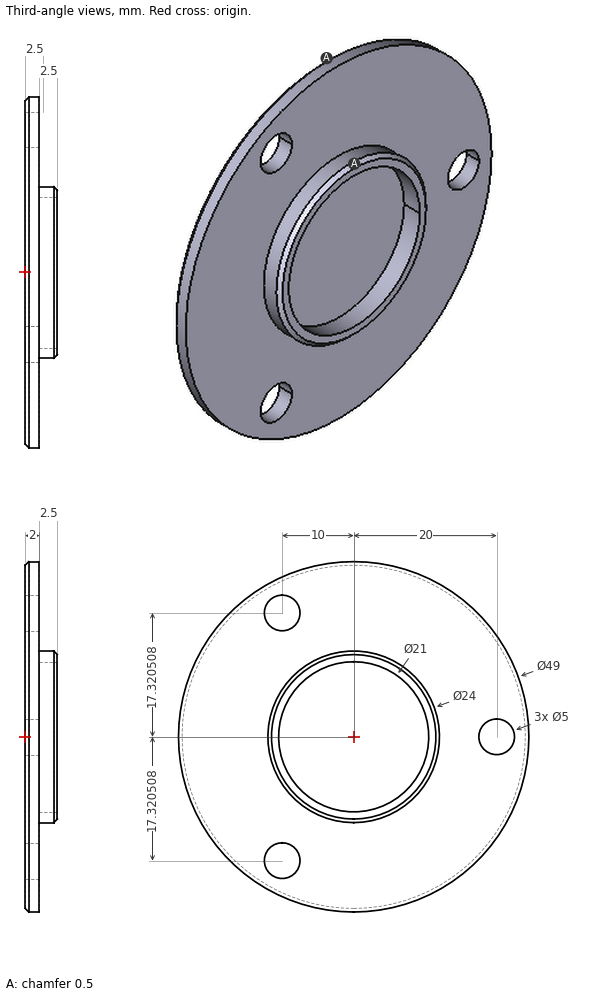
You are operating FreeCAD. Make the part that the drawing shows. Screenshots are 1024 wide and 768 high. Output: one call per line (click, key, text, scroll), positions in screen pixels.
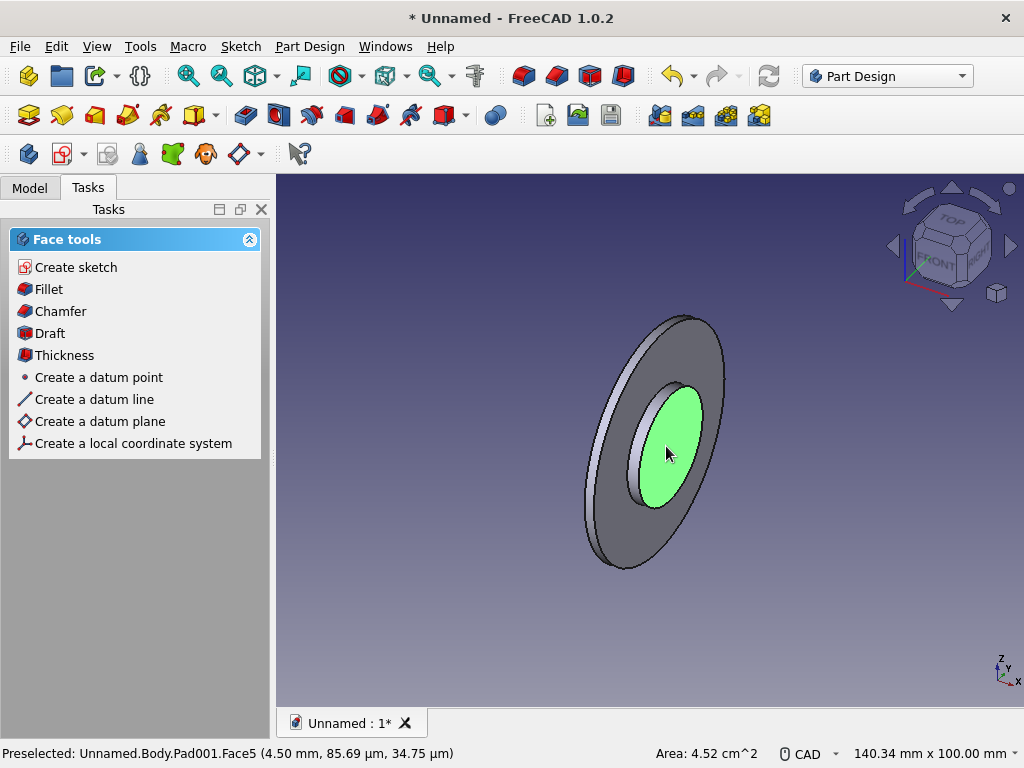
click(62, 154)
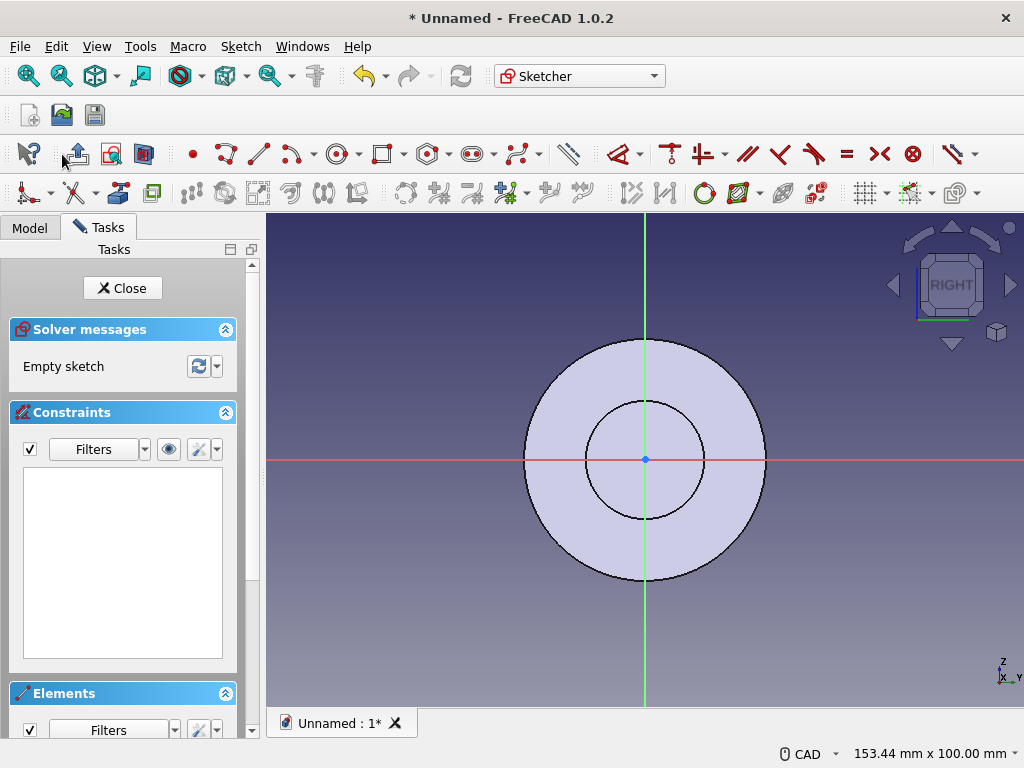
scroll(685, 460, up, 5)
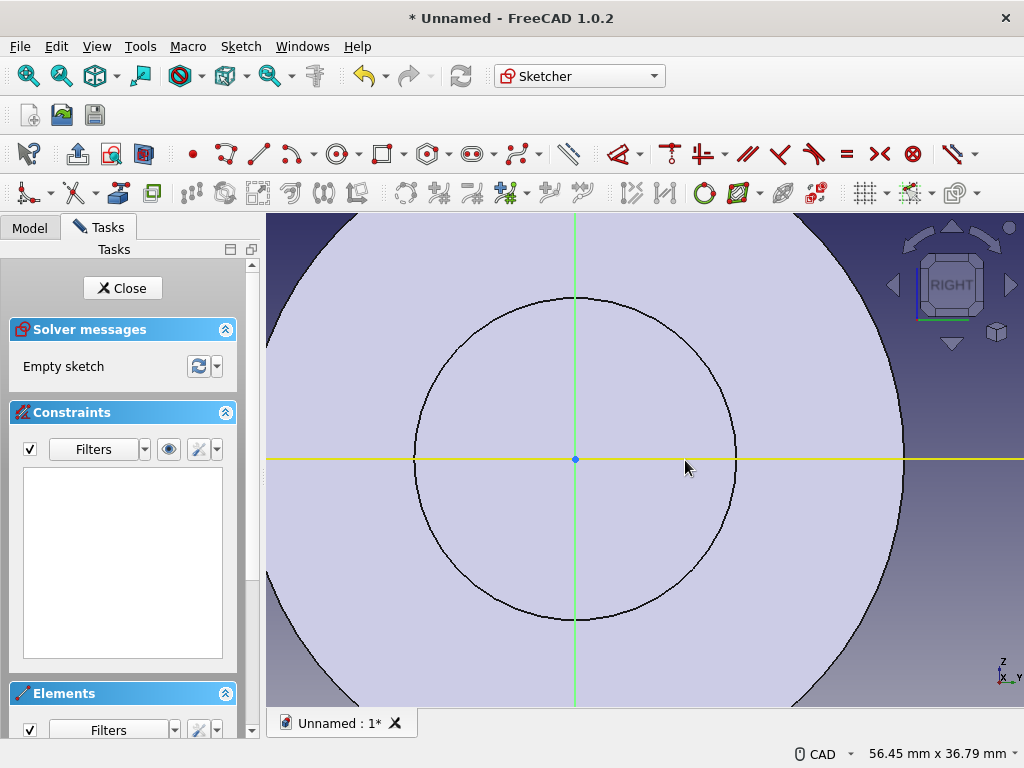
click(336, 154)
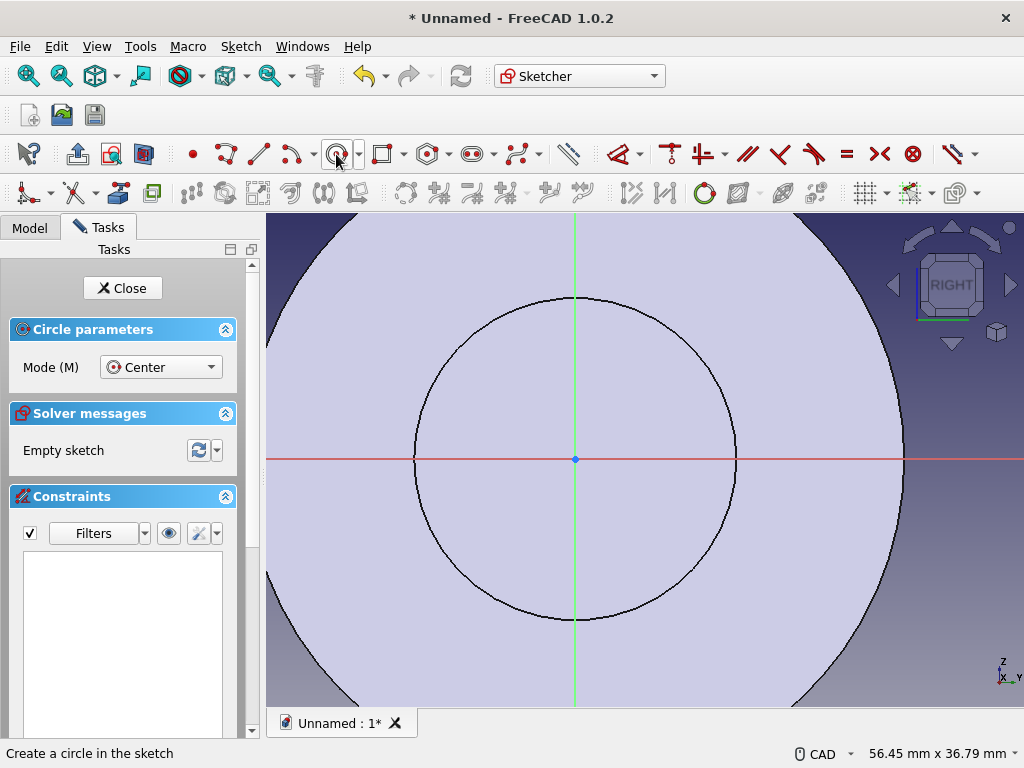
click(575, 459)
click(675, 359)
key(Escape)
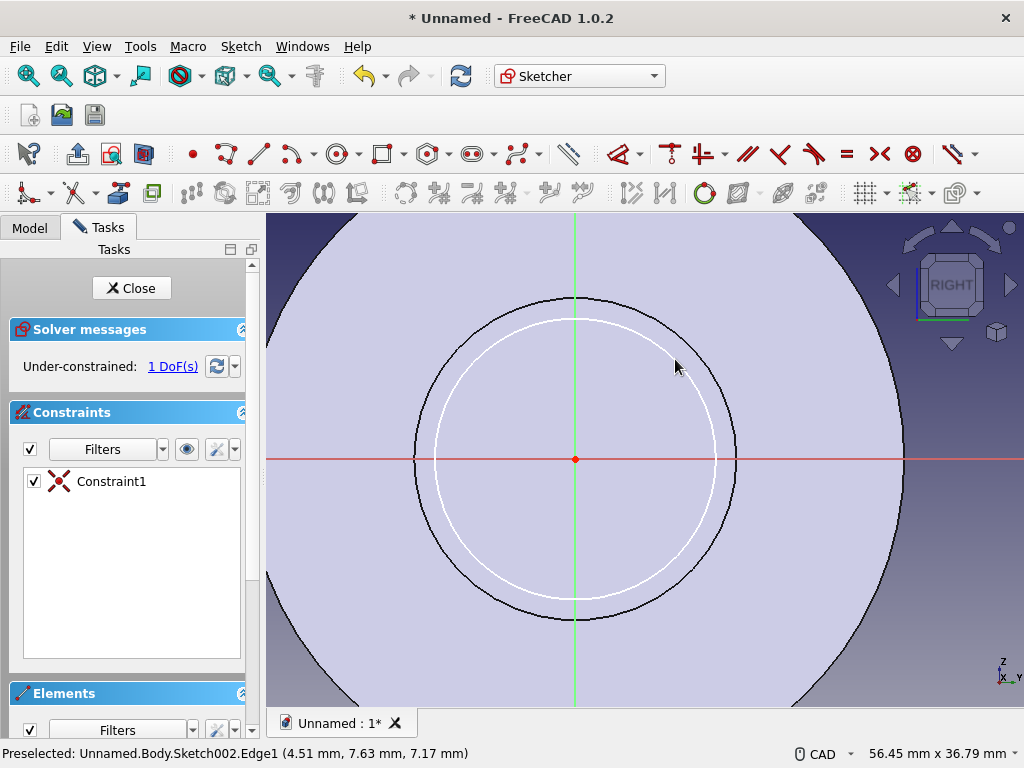
click(618, 154)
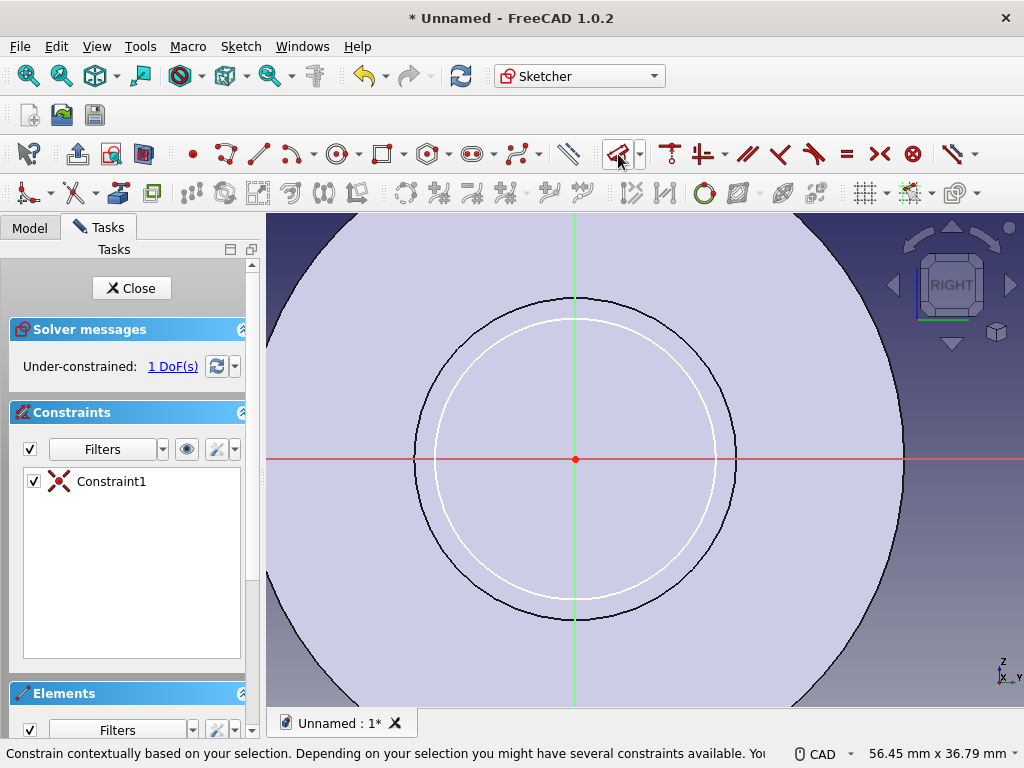
click(674, 359)
click(696, 336)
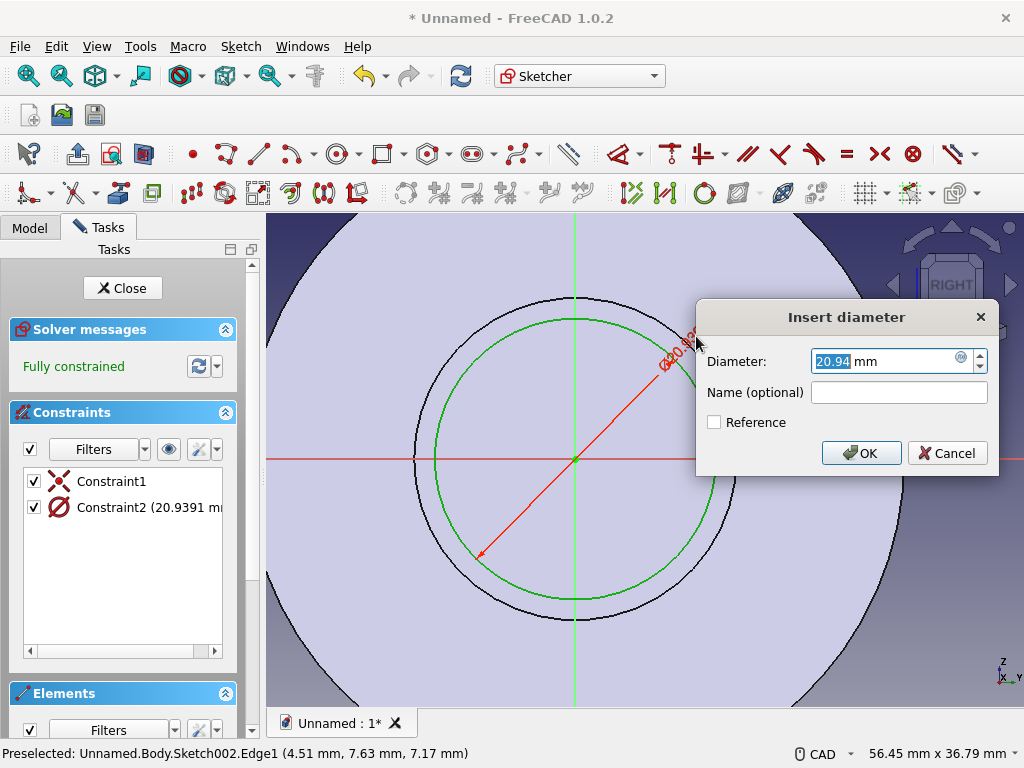
text(21)
key(Return)
key(Escape)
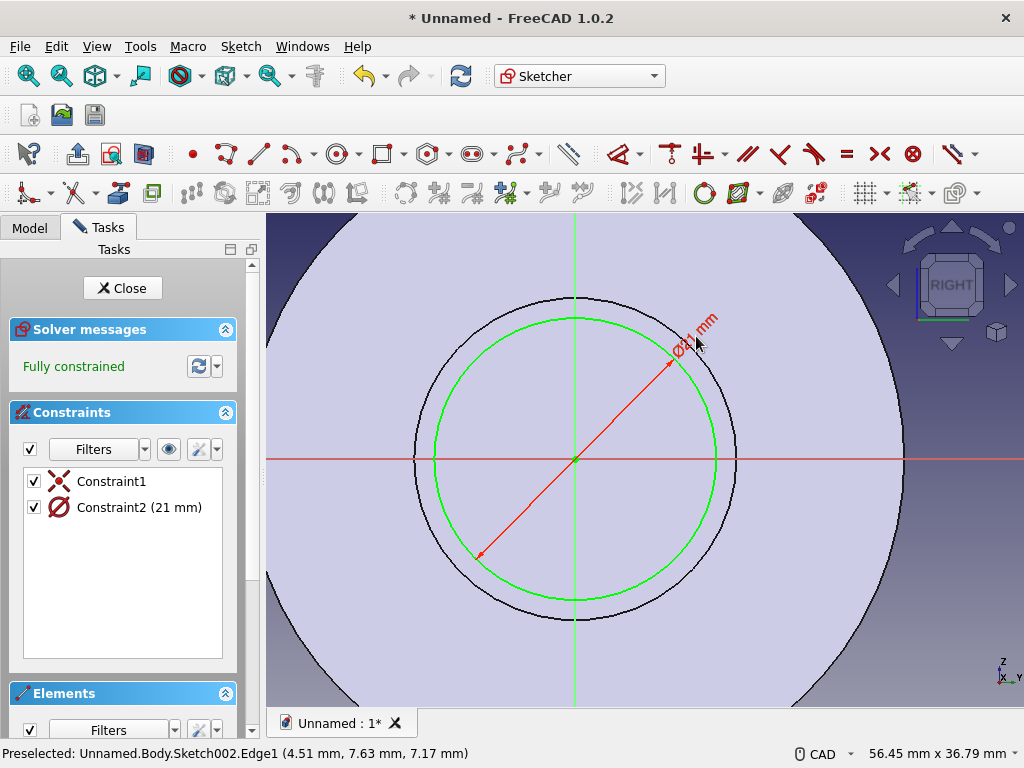
click(123, 288)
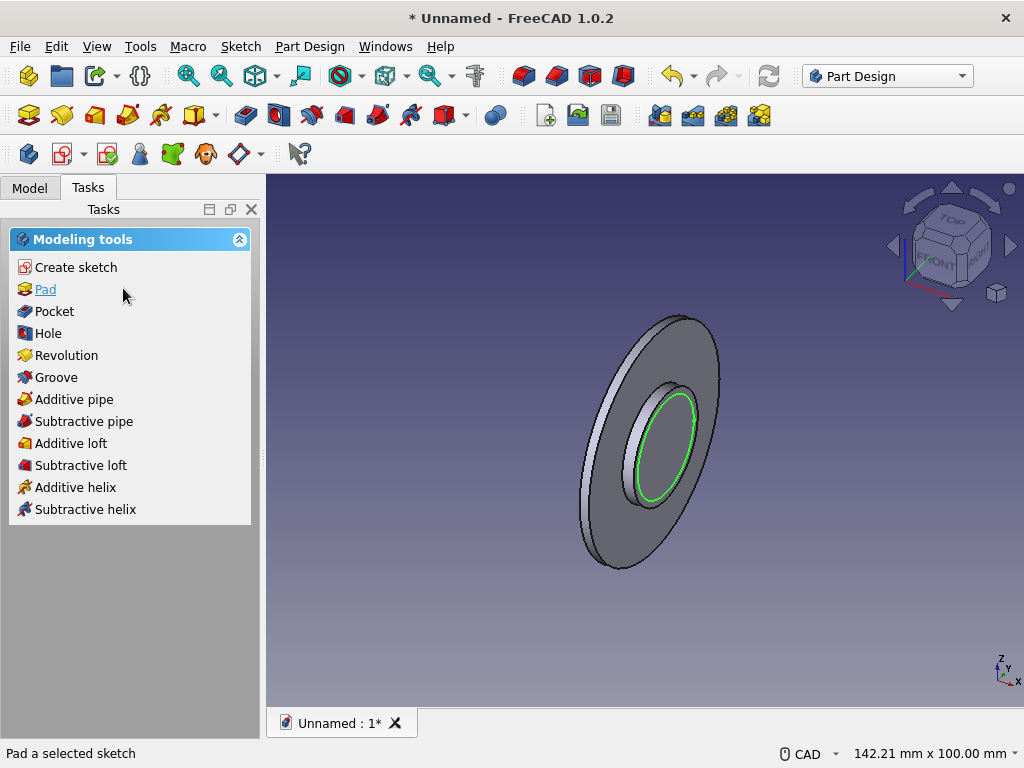
click(246, 116)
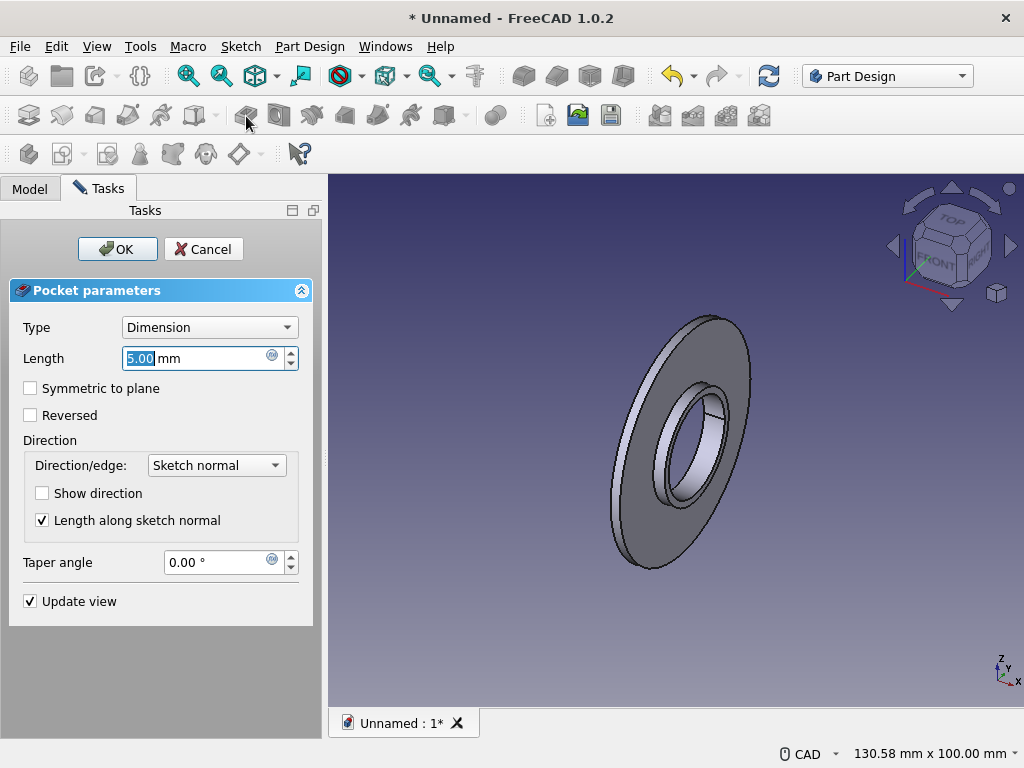
click(210, 328)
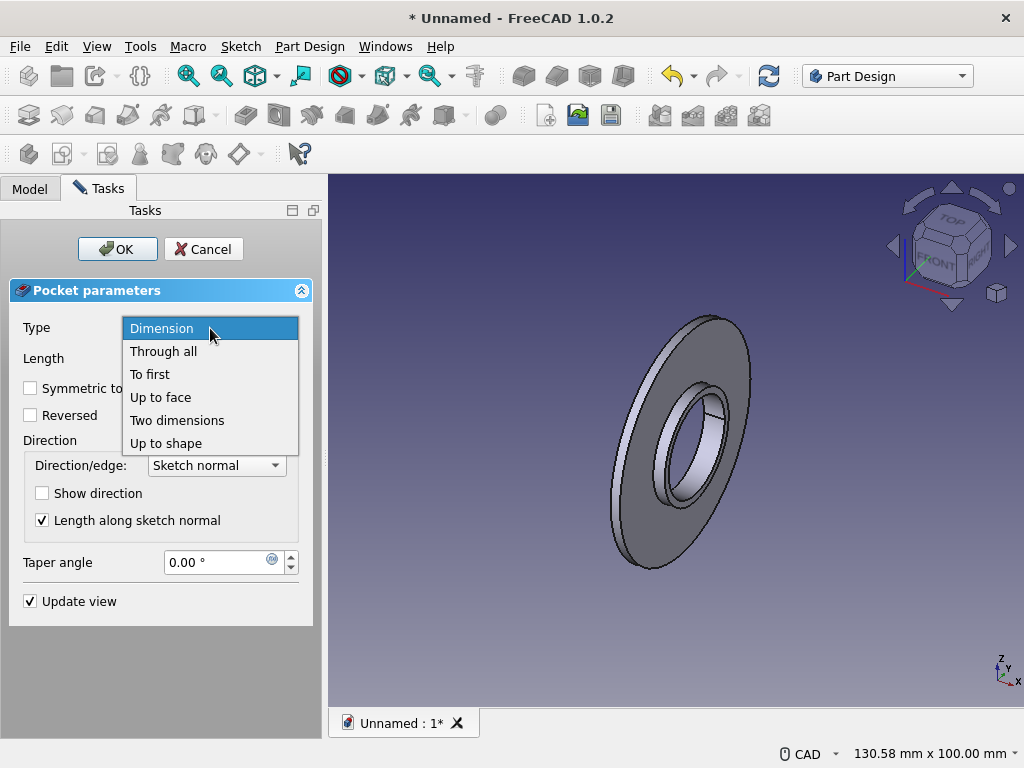
click(208, 420)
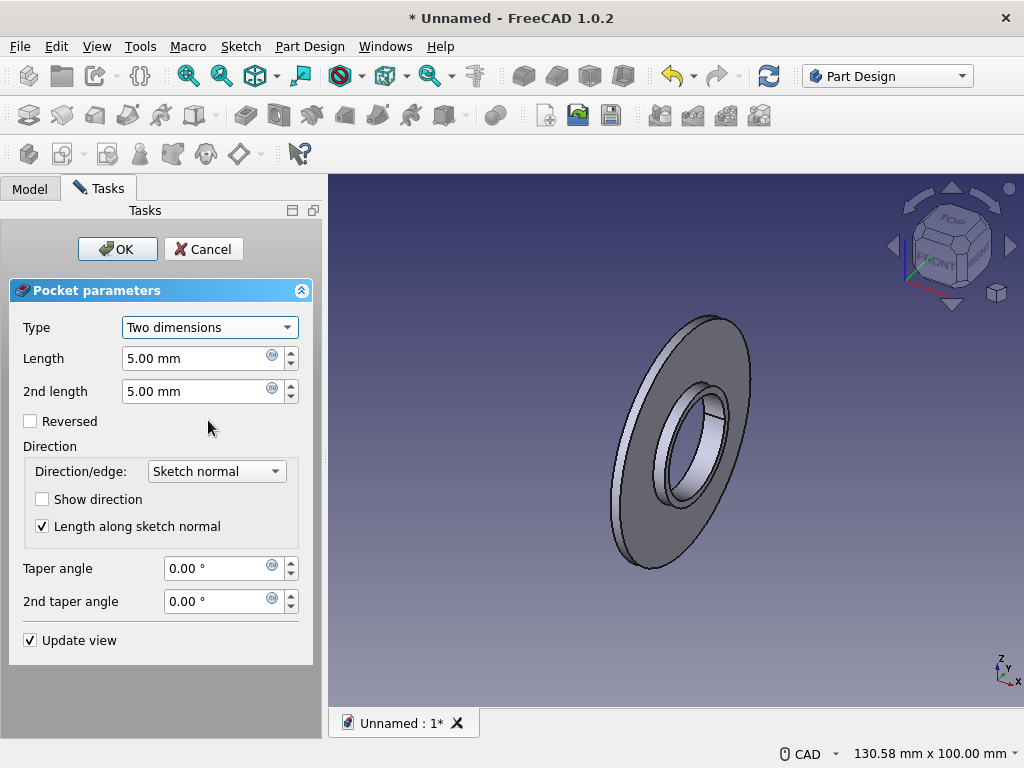
triple_click(204, 358)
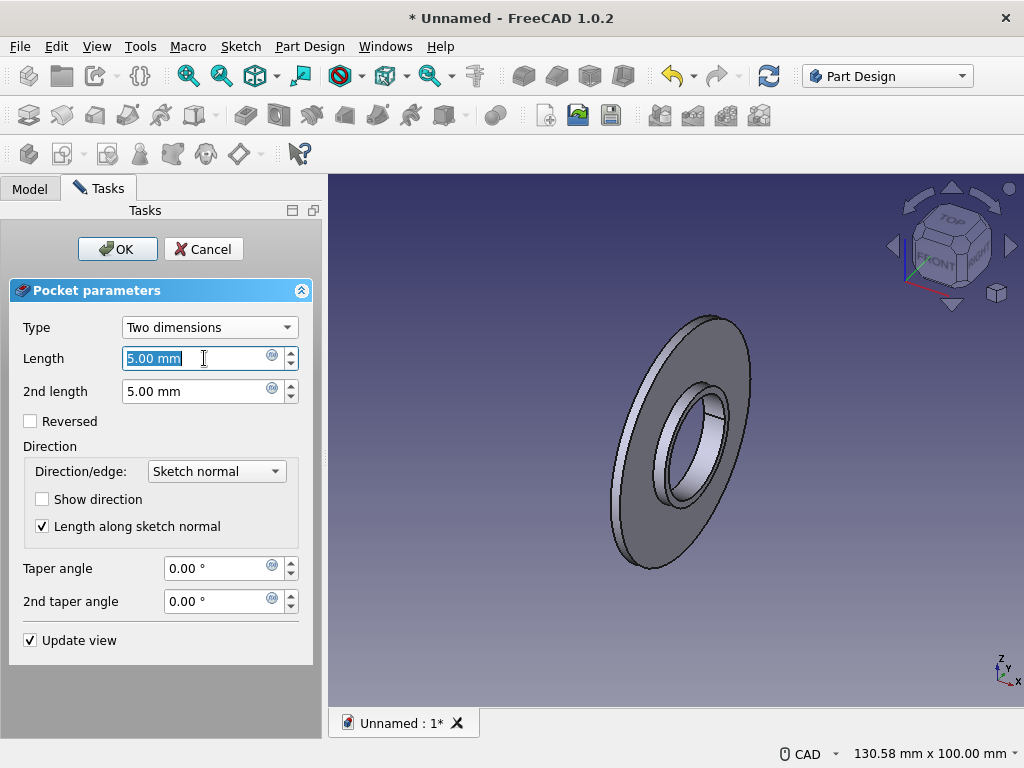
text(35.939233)
key(Tab)